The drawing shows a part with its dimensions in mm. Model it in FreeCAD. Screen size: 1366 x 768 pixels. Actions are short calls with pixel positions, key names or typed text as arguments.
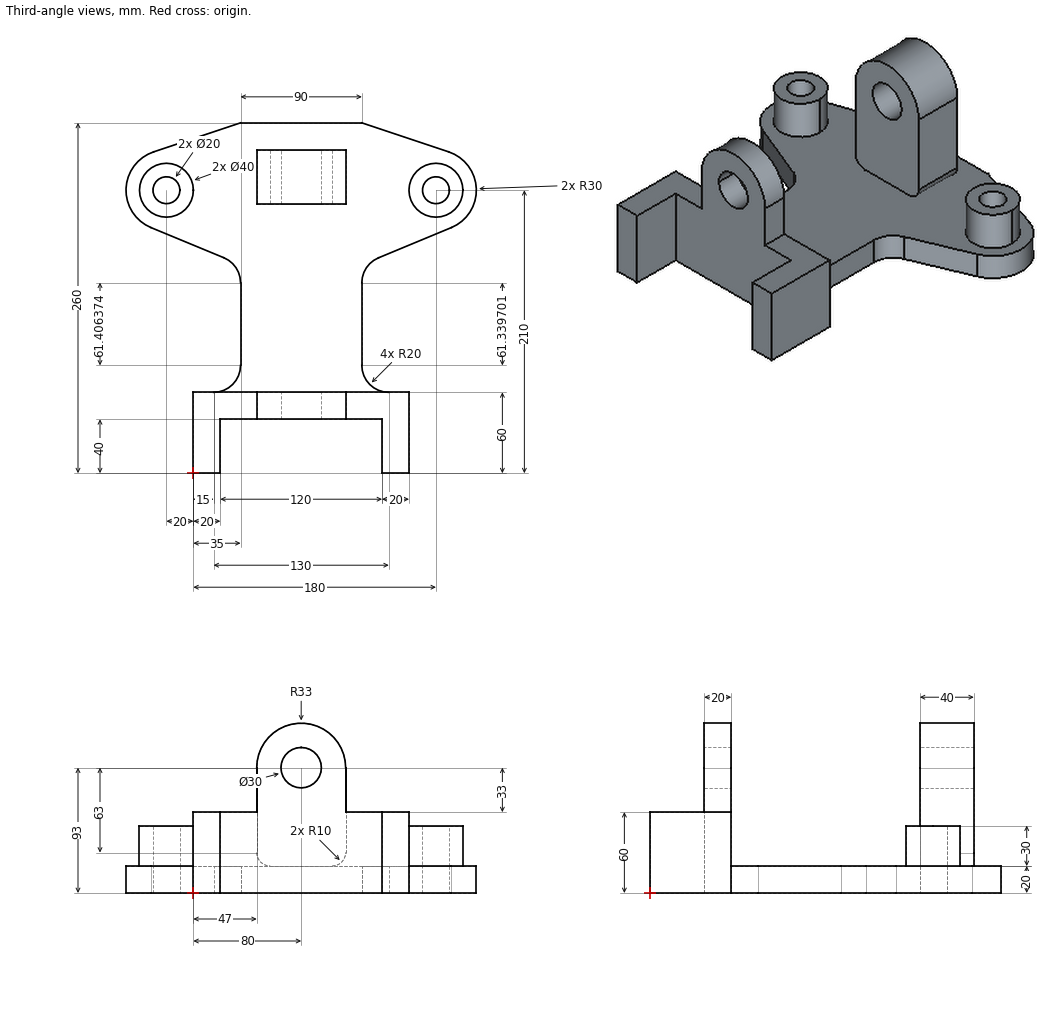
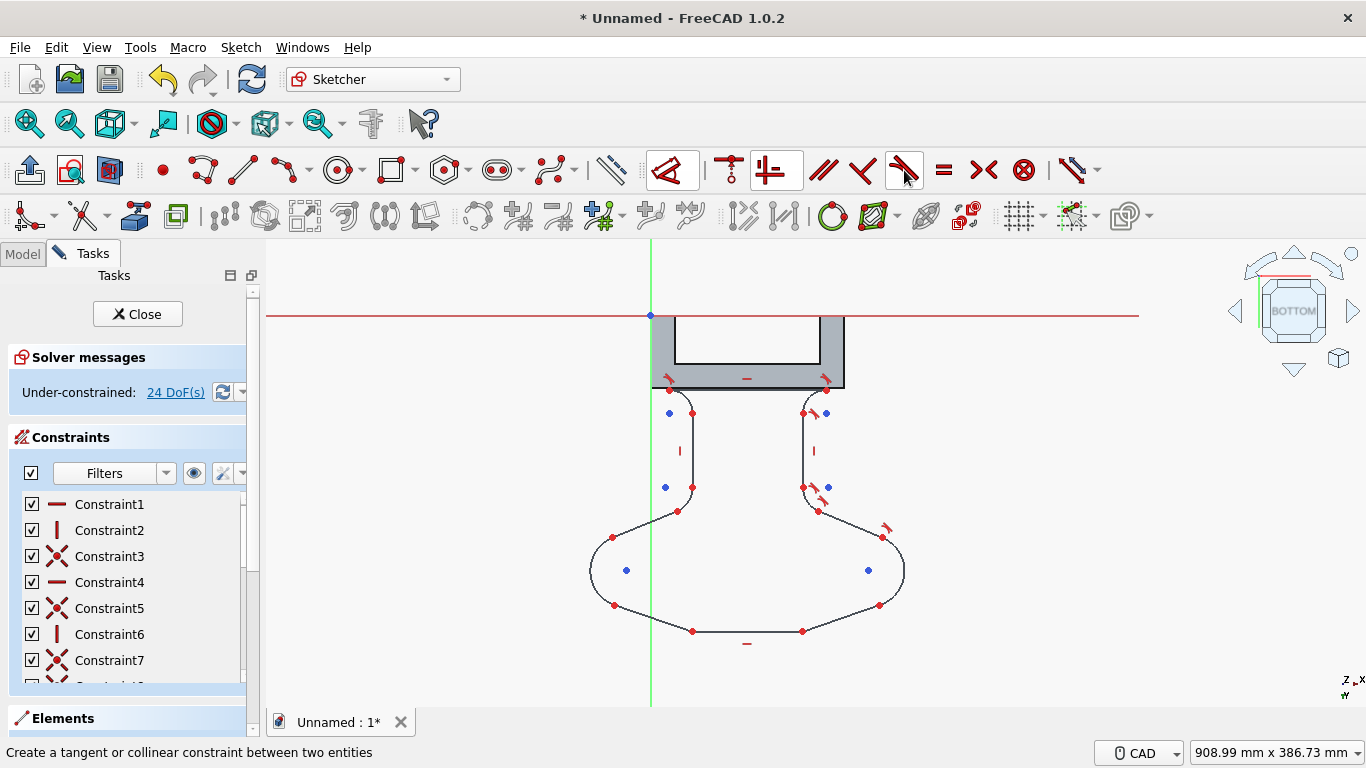
click(856, 613)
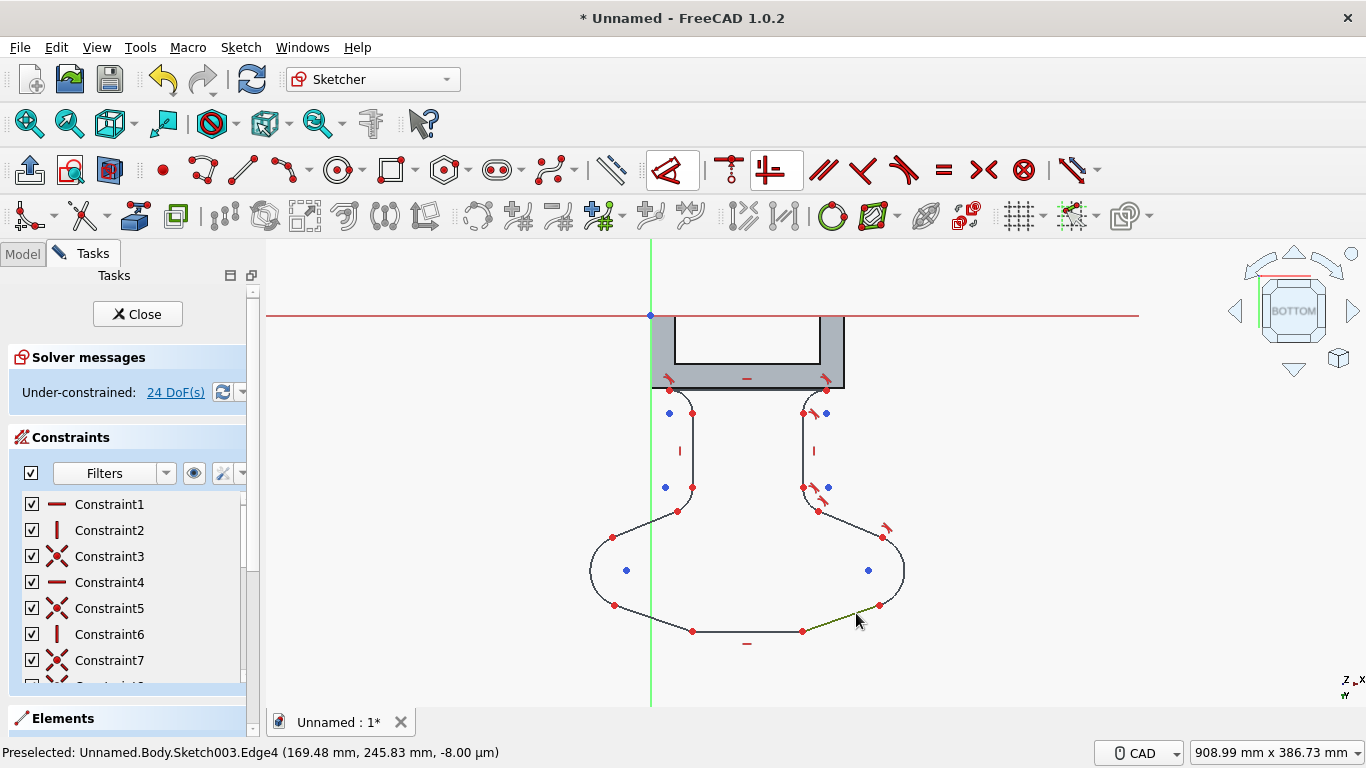
click(900, 589)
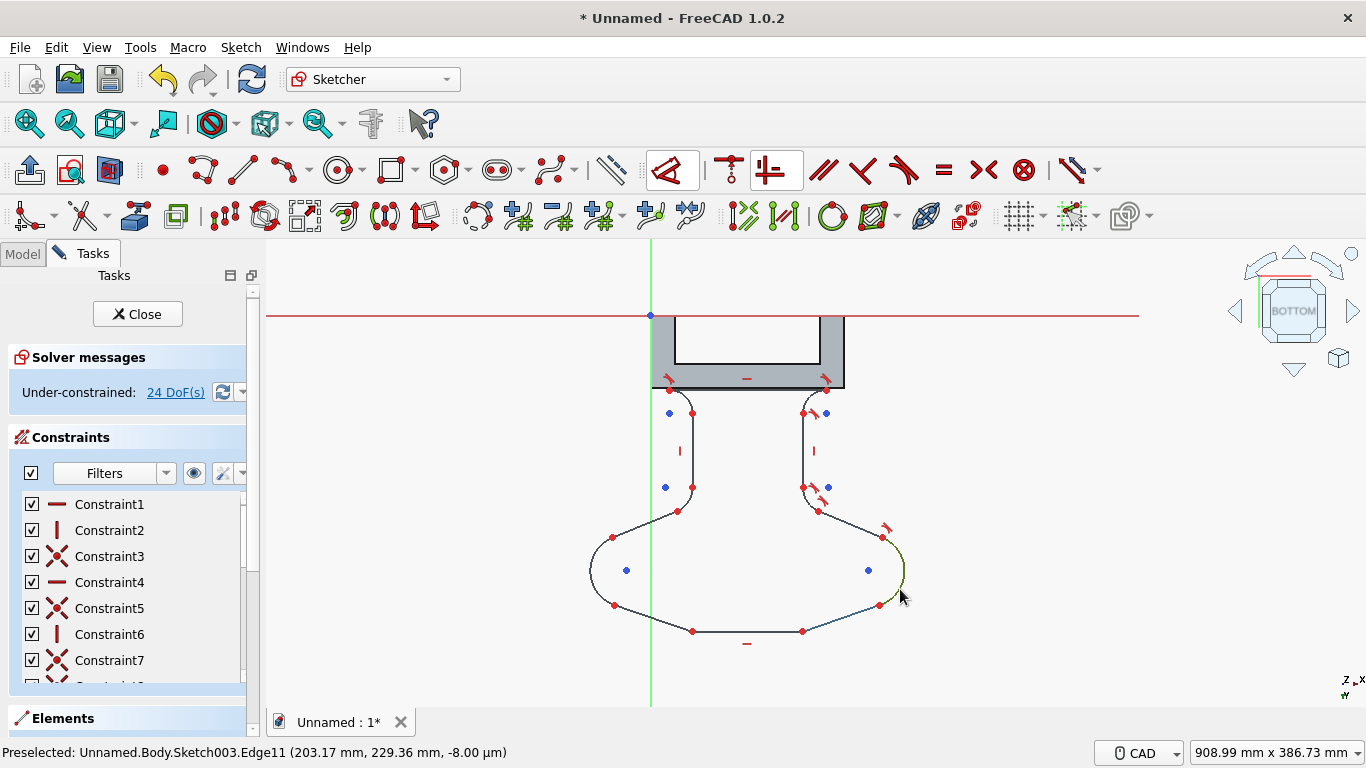
click(904, 170)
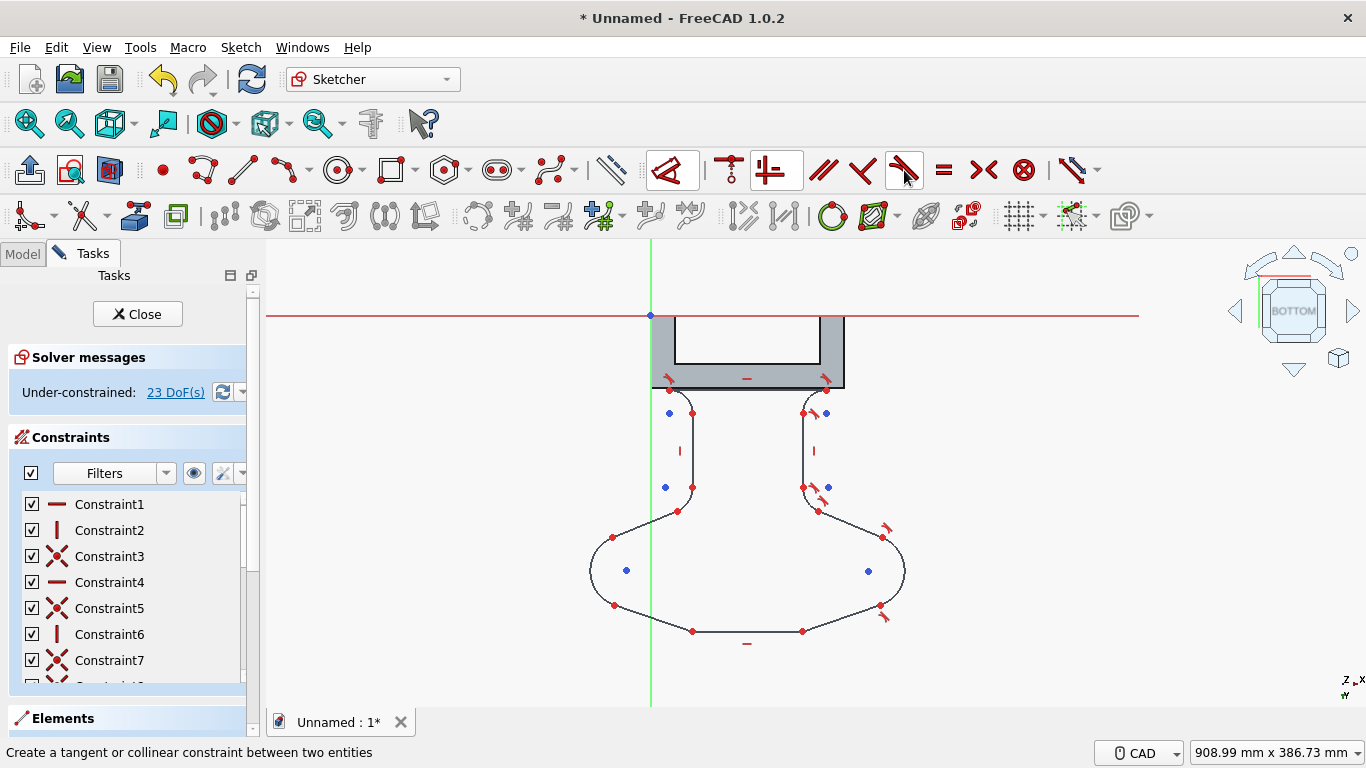
click(669, 624)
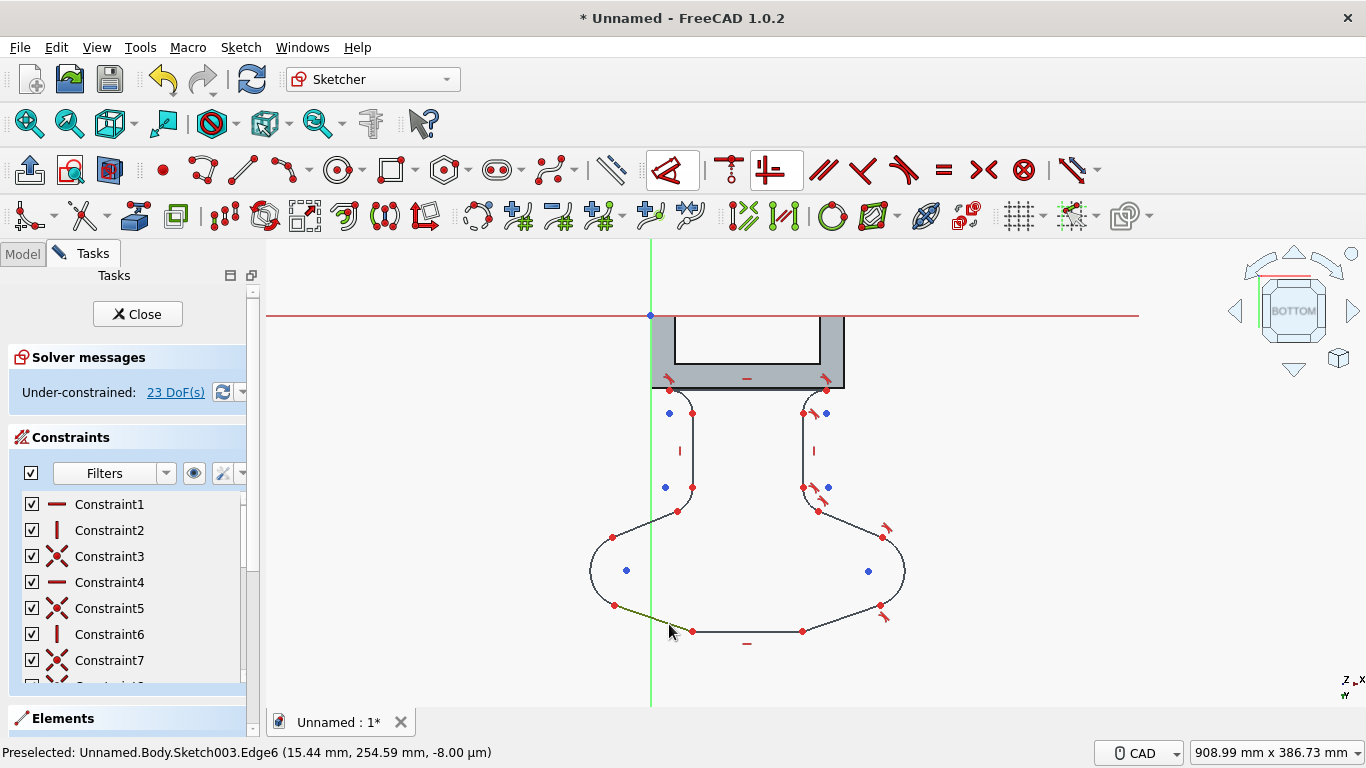
click(594, 556)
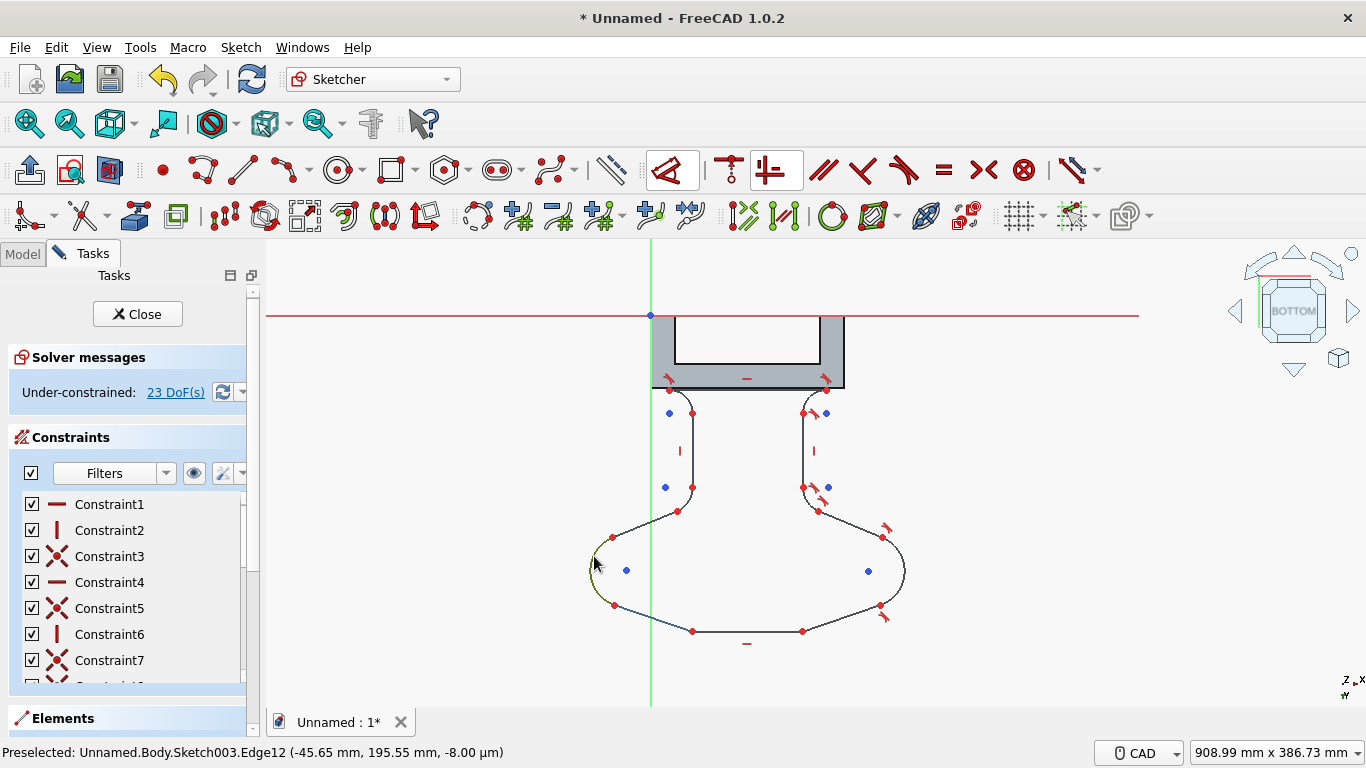
click(904, 170)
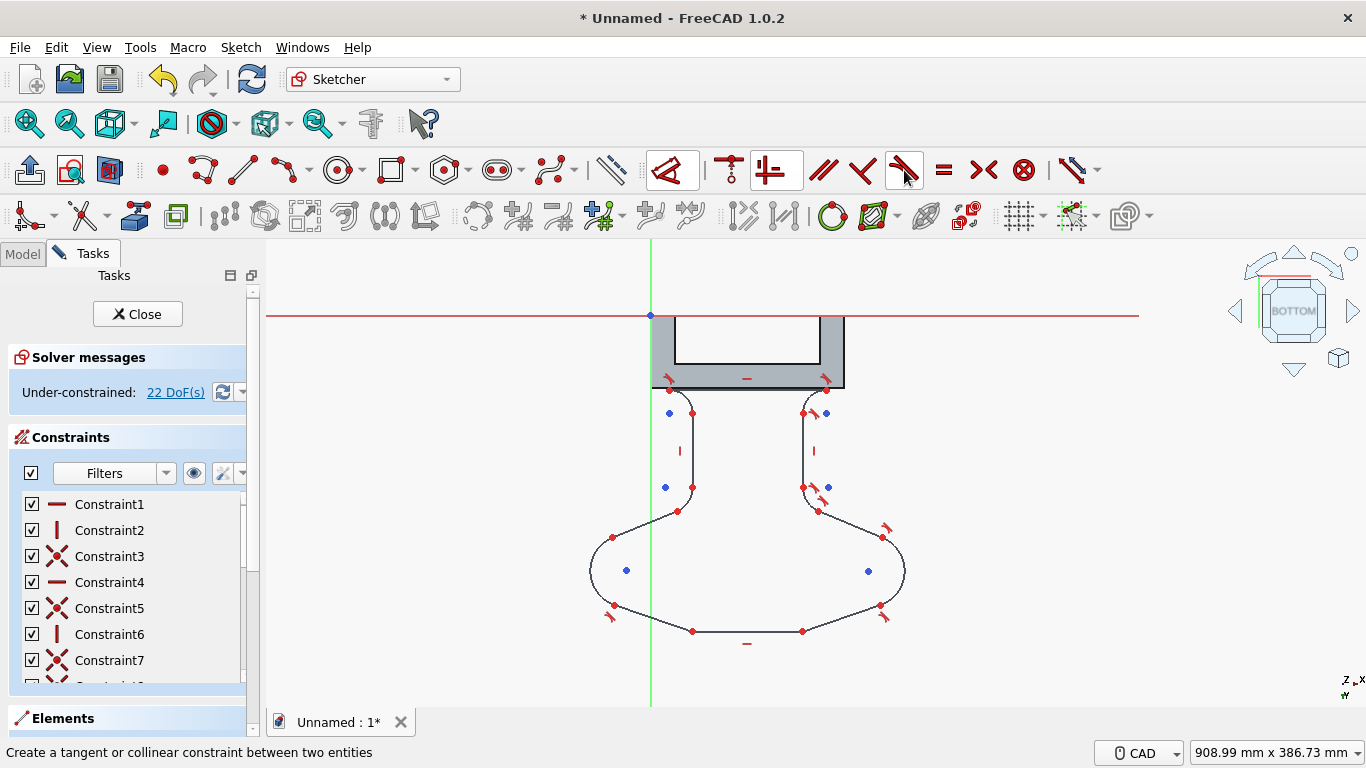
click(632, 530)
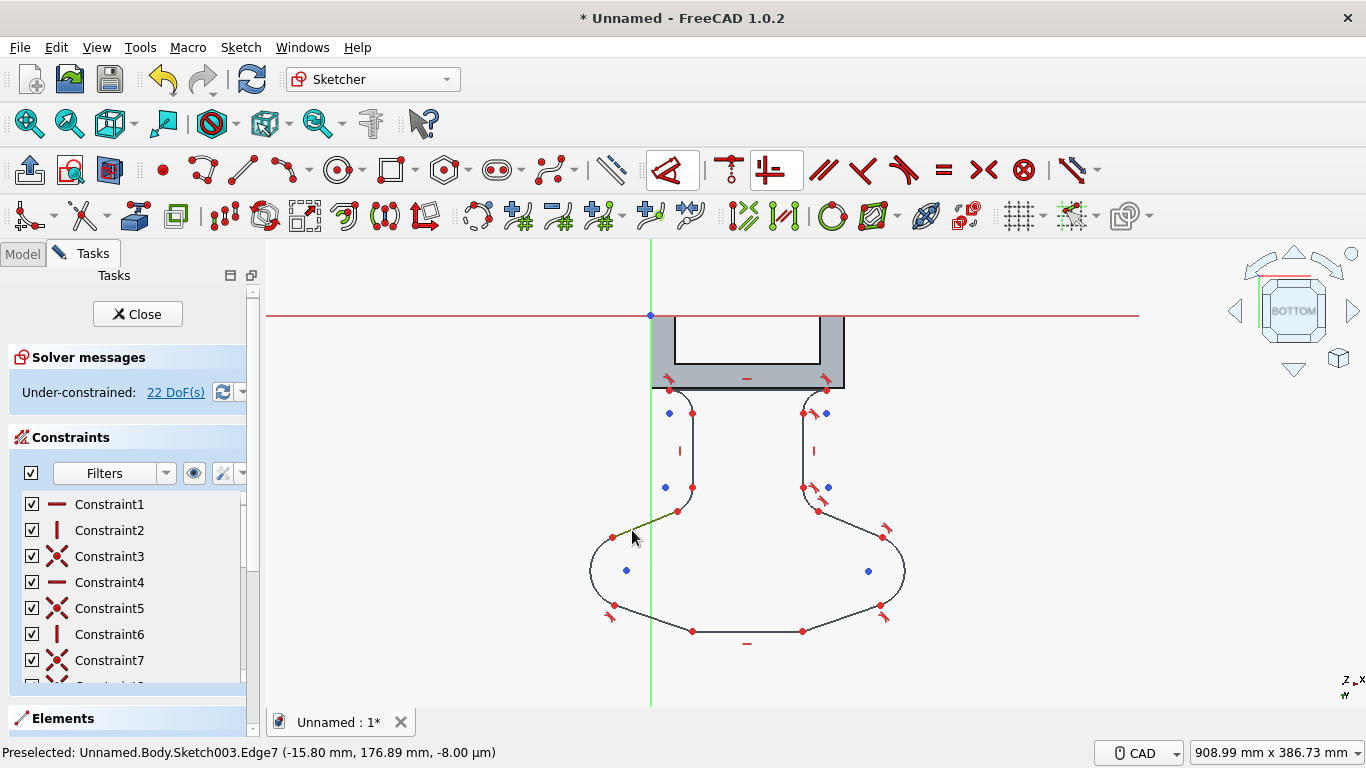
click(594, 556)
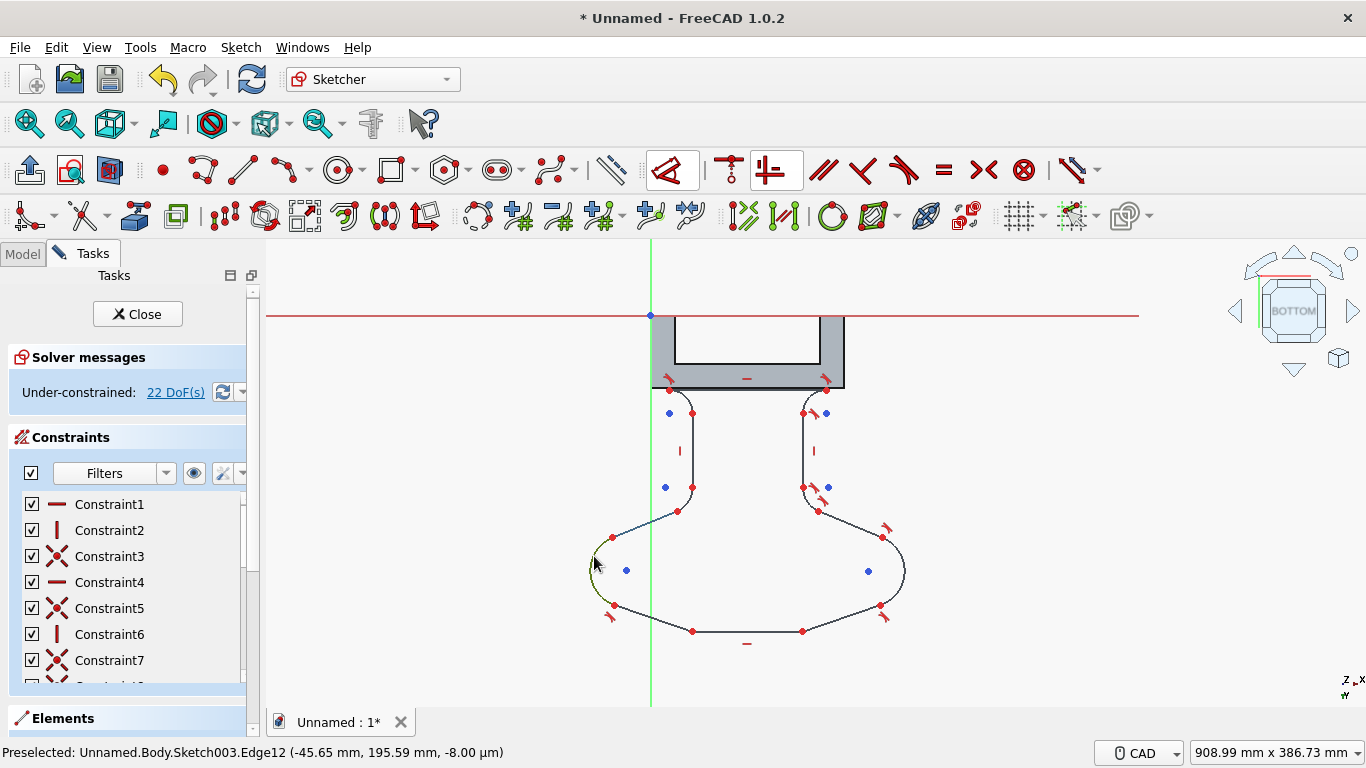
key(t)